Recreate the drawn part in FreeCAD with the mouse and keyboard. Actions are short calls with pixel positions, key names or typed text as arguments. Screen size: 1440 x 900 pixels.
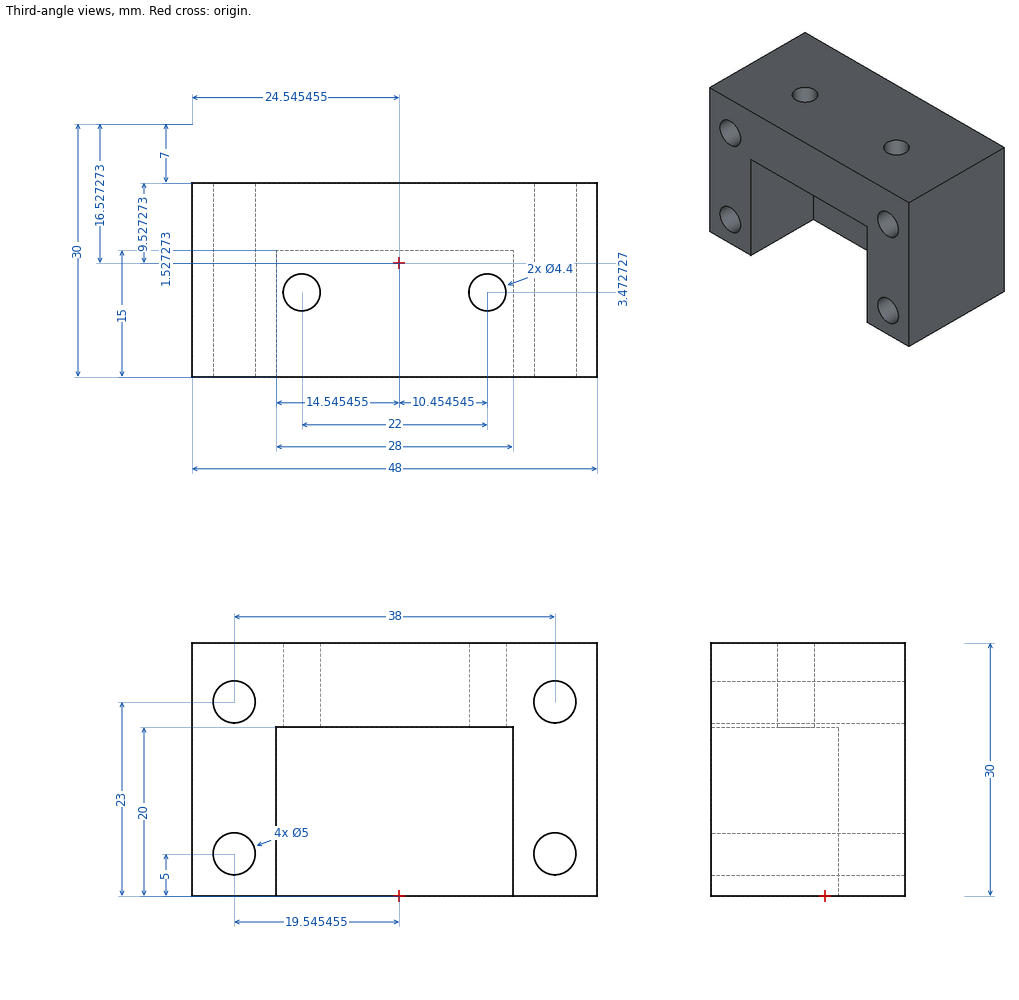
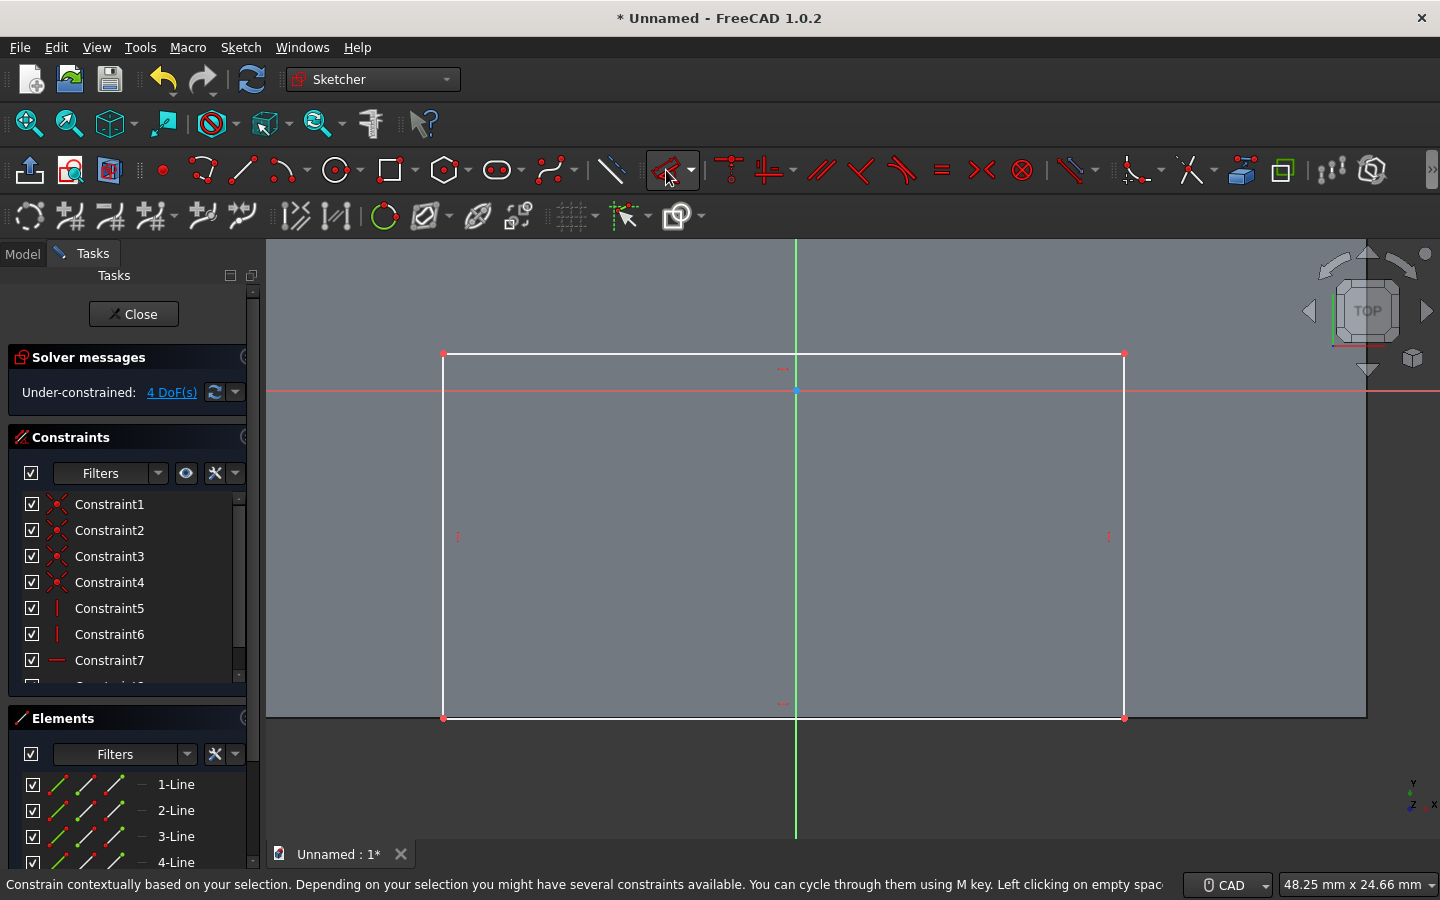
click(443, 463)
click(409, 536)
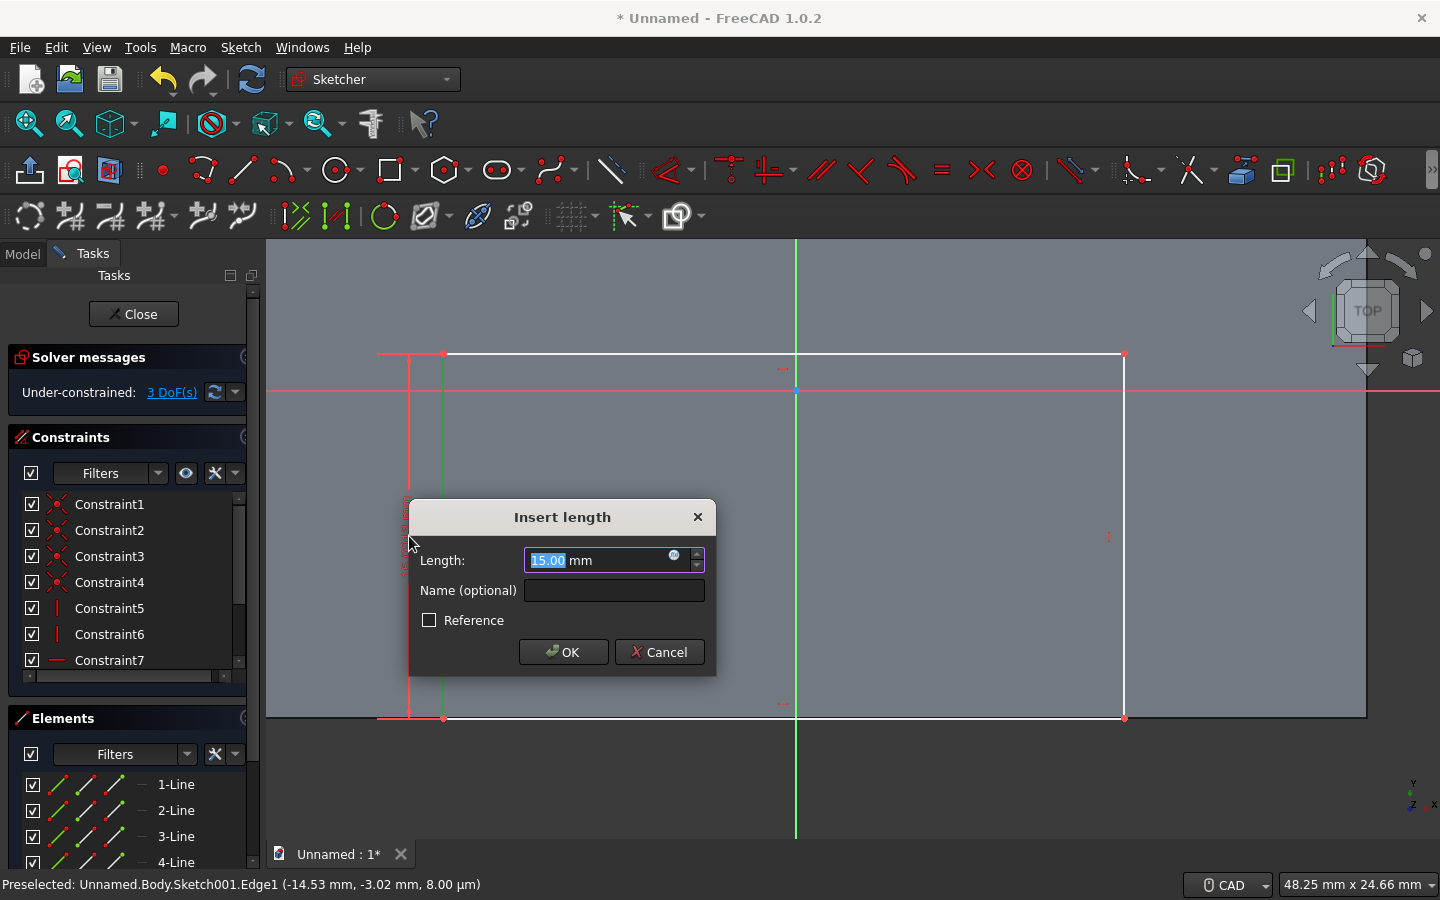
text(15)
key(Return)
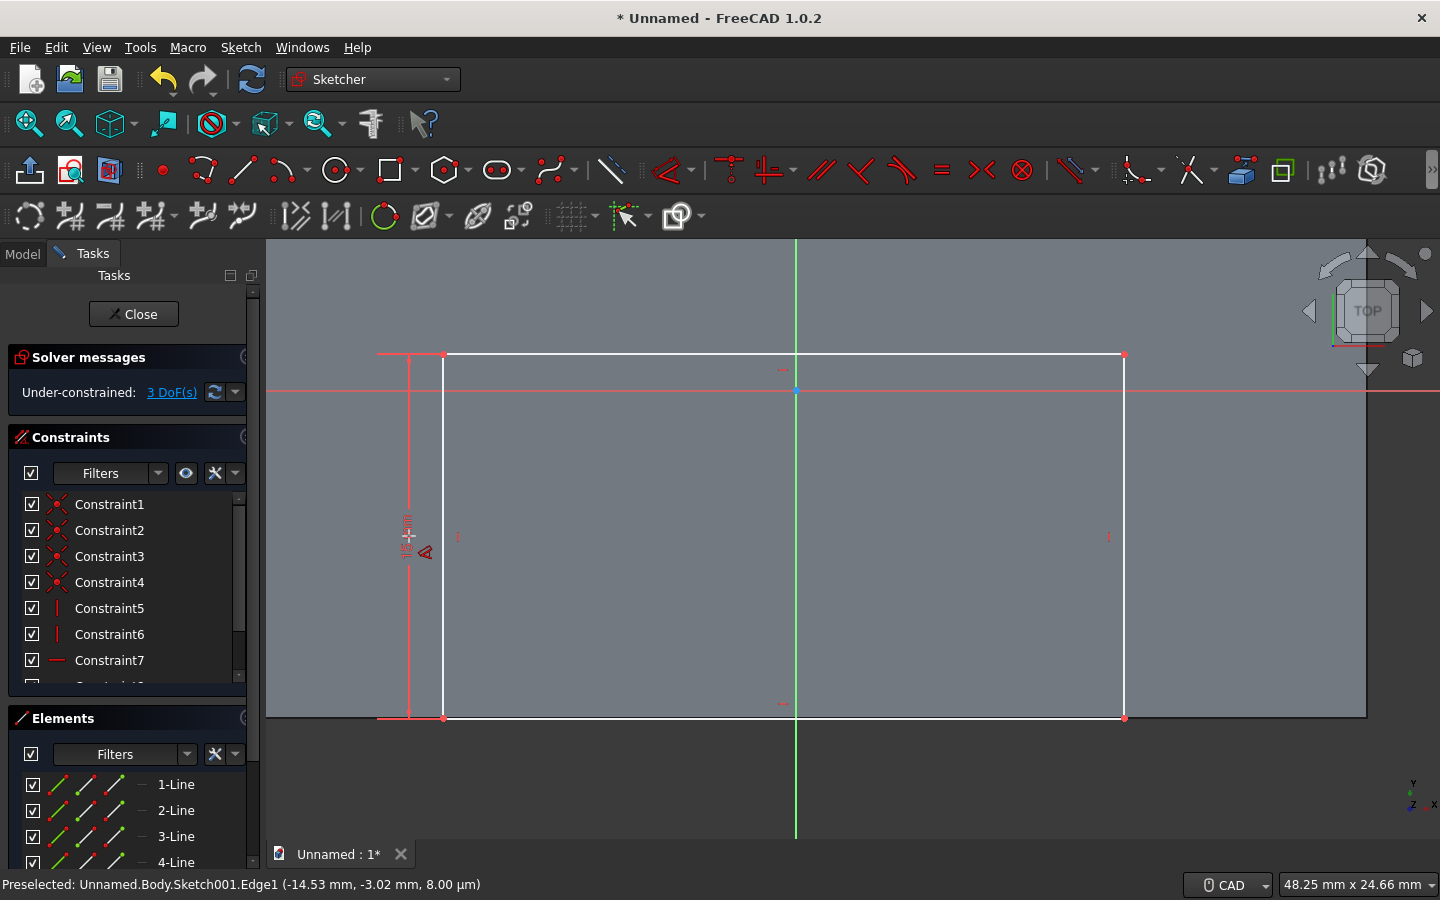
click(647, 719)
click(627, 753)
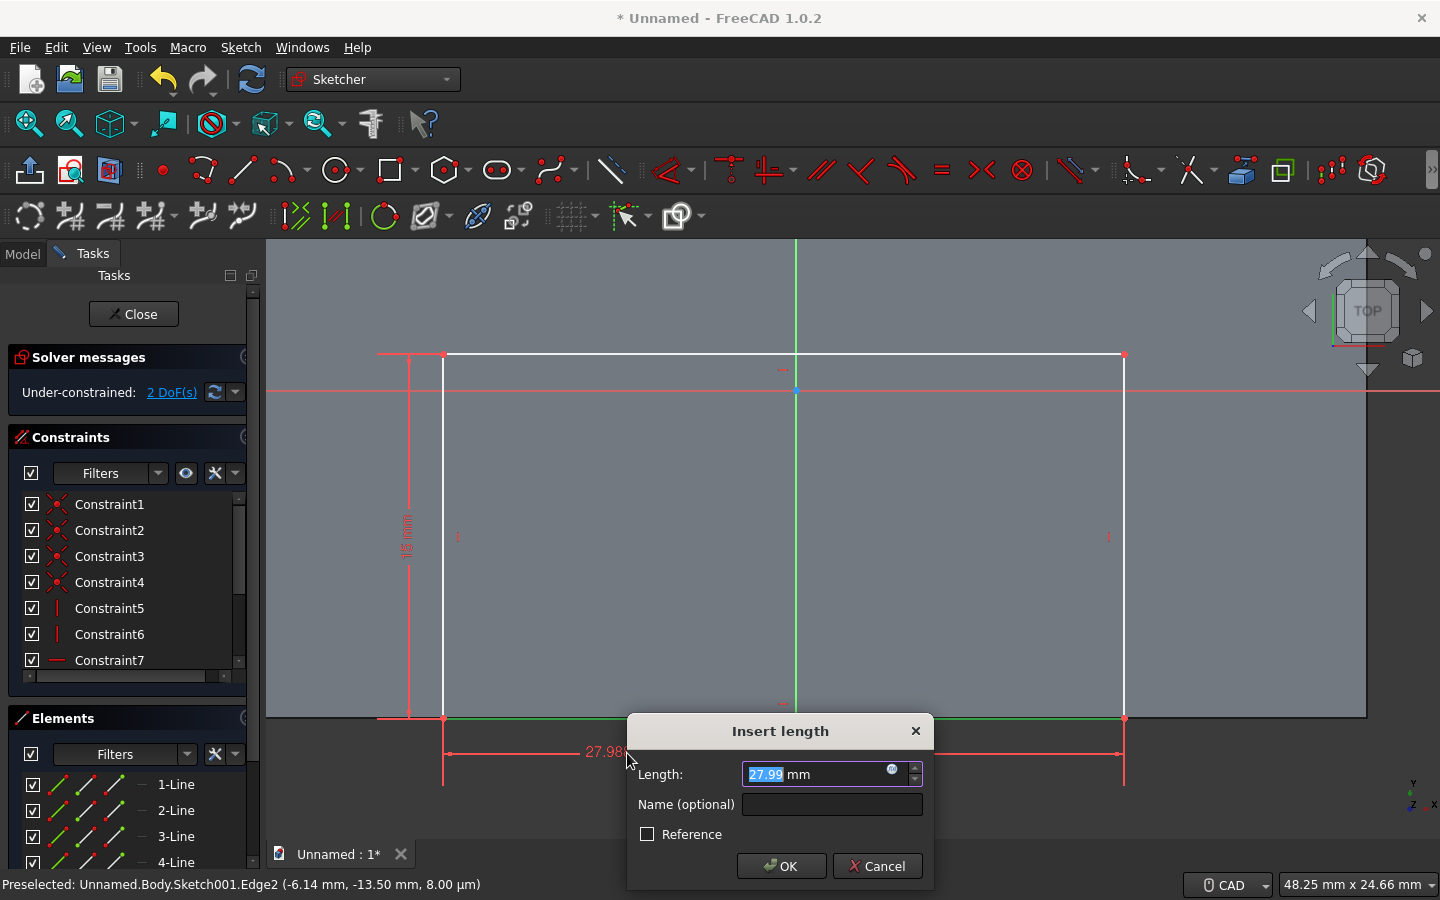
text(28)
key(Return)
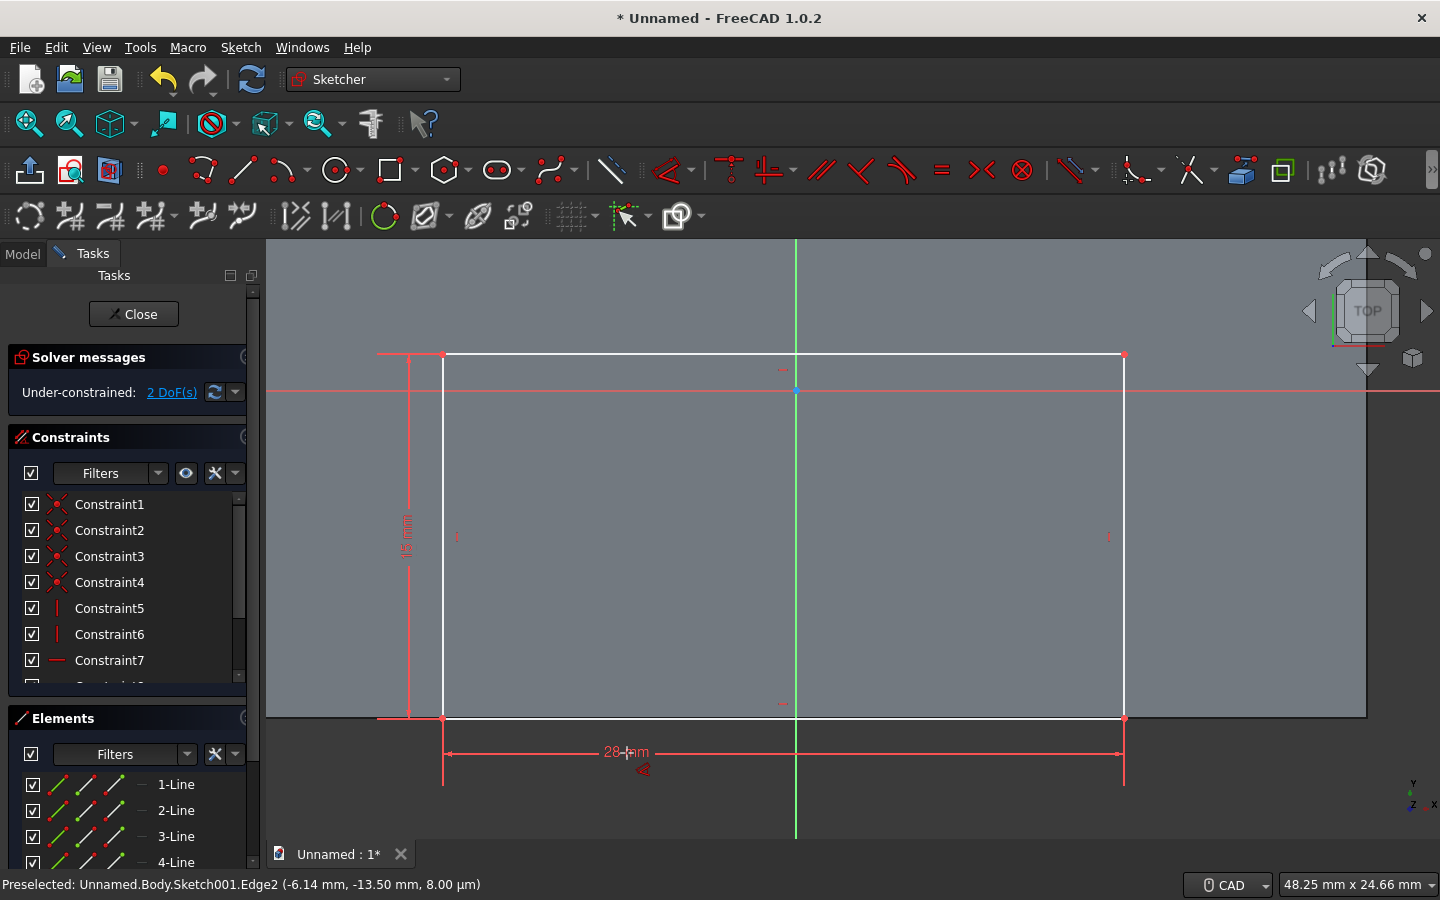
click(443, 354)
click(409, 372)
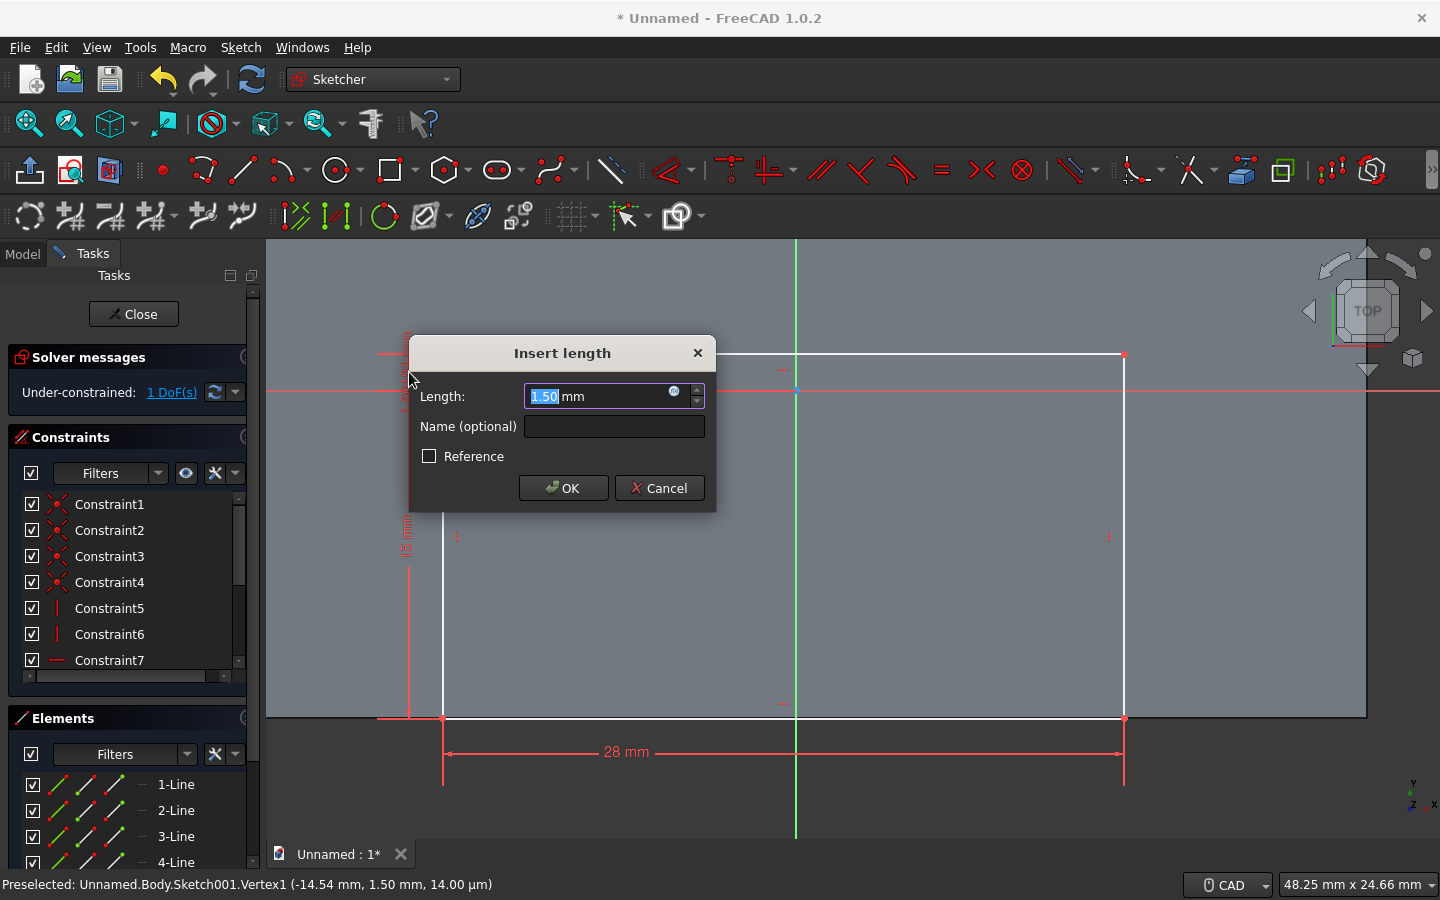
text(1.527273)
key(Return)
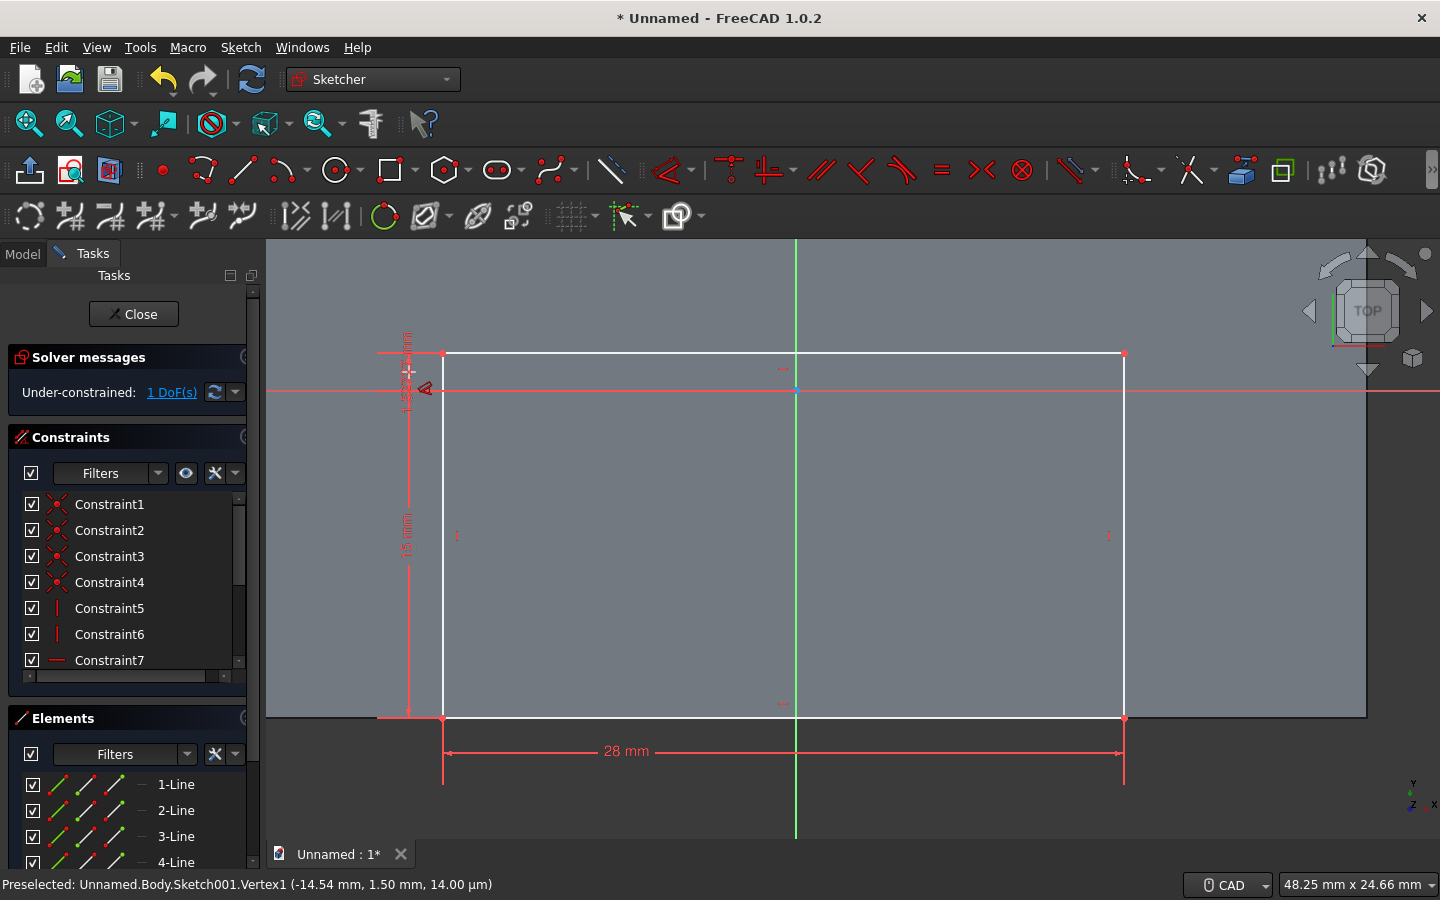
click(443, 353)
click(620, 319)